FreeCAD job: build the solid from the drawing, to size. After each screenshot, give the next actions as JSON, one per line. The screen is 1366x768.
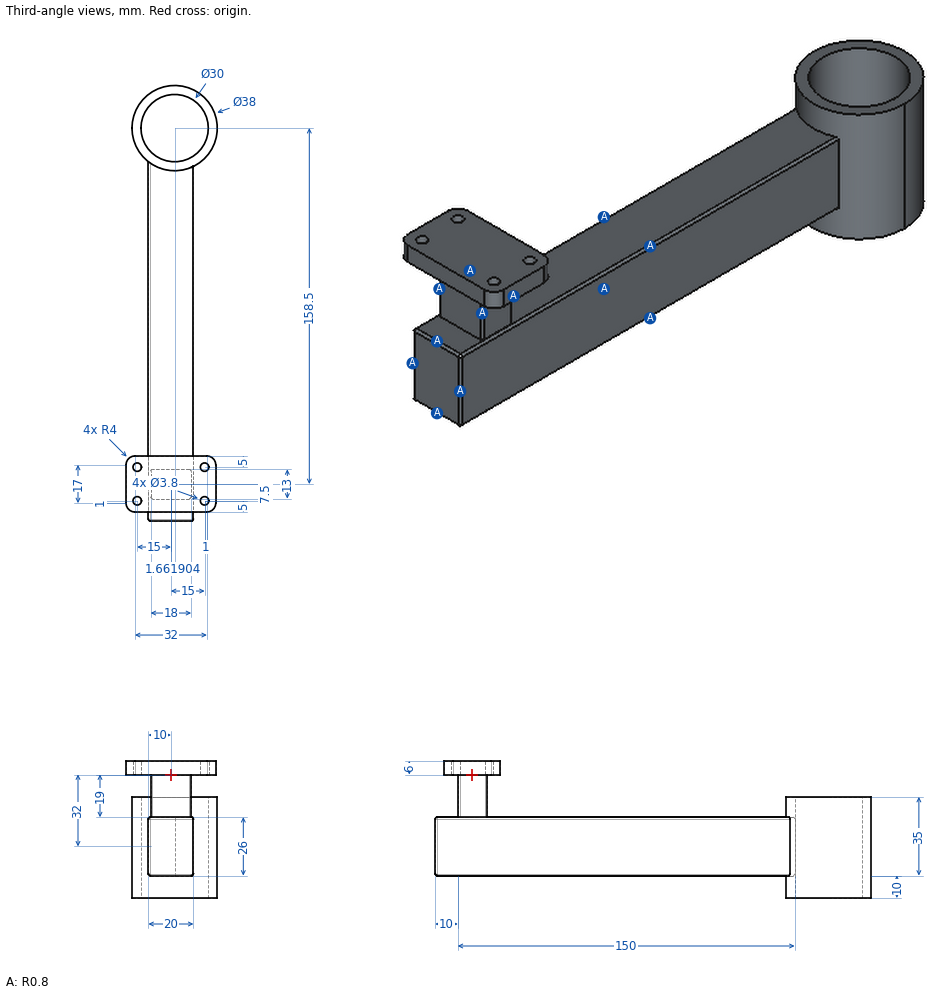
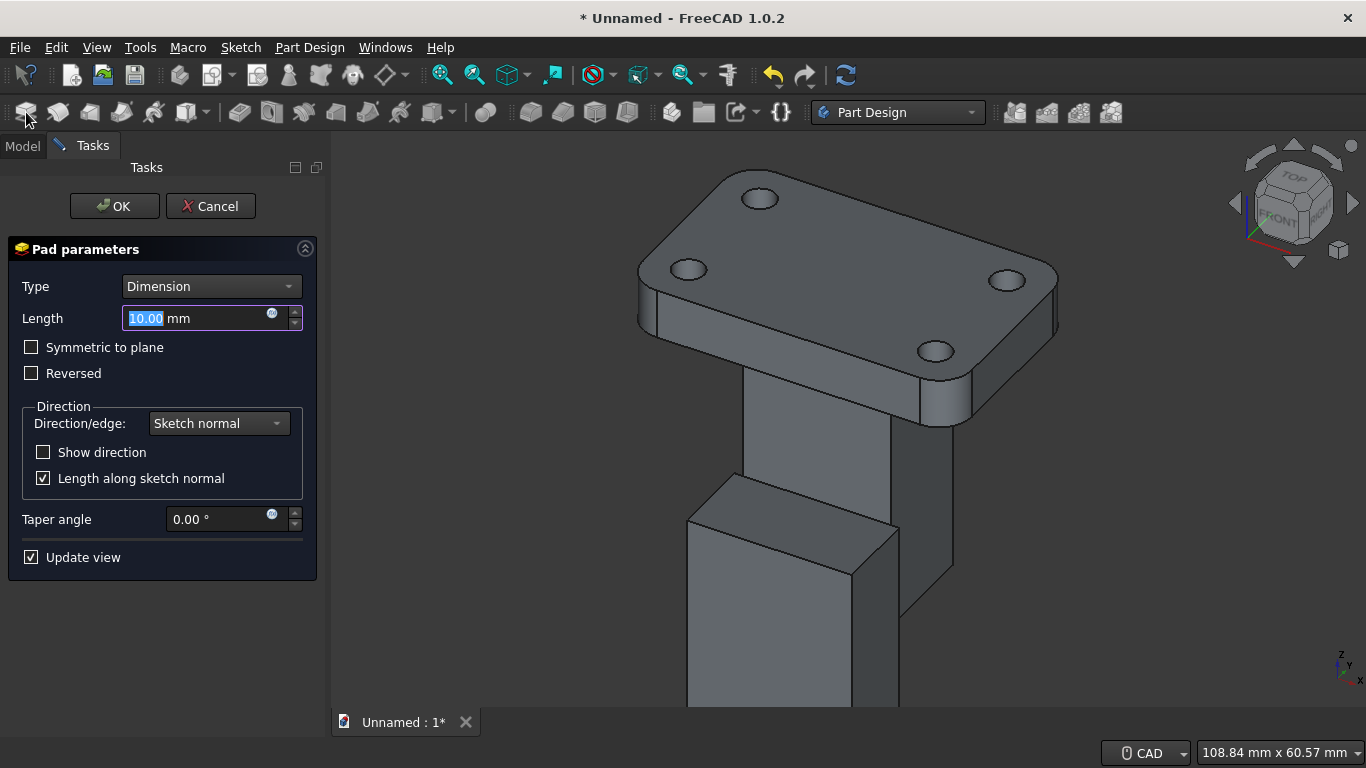
{"action": "left_click", "coordinate": [212, 286]}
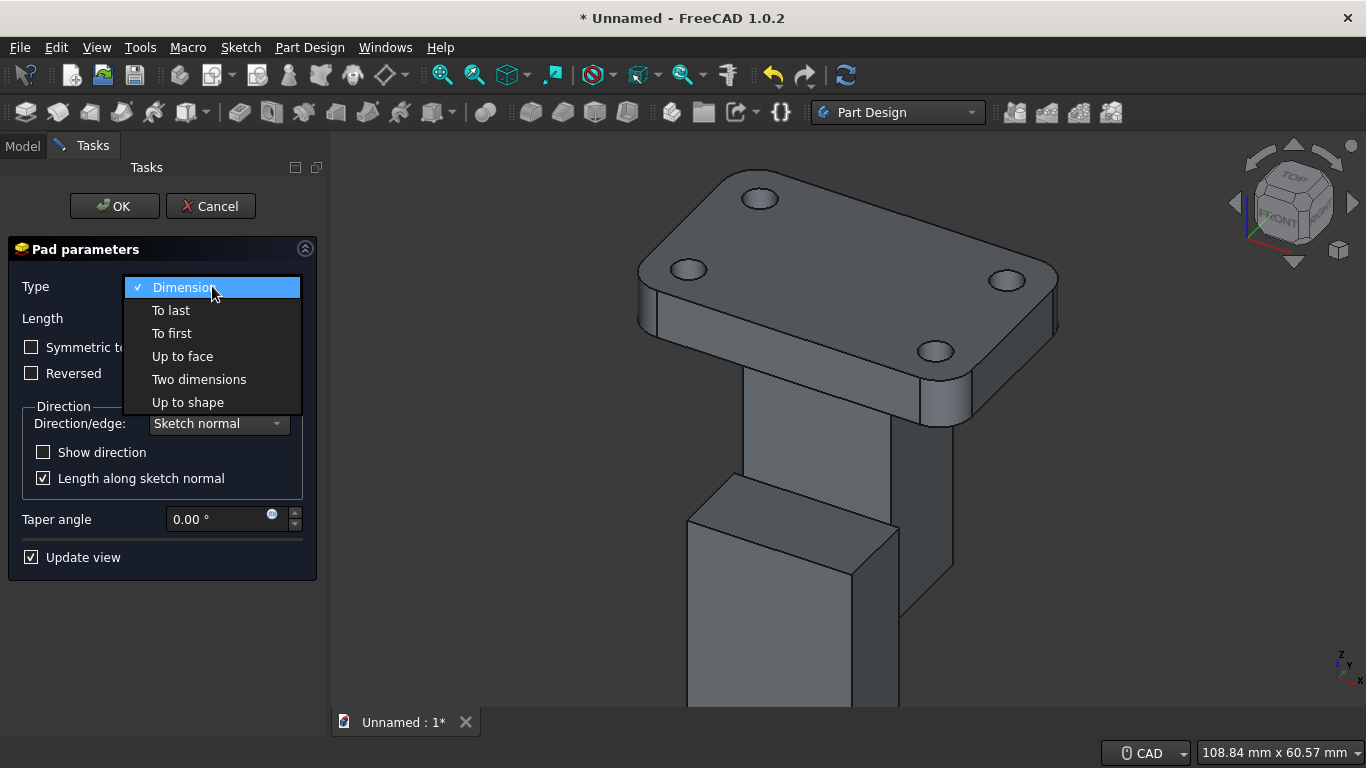
{"action": "left_click", "coordinate": [212, 380]}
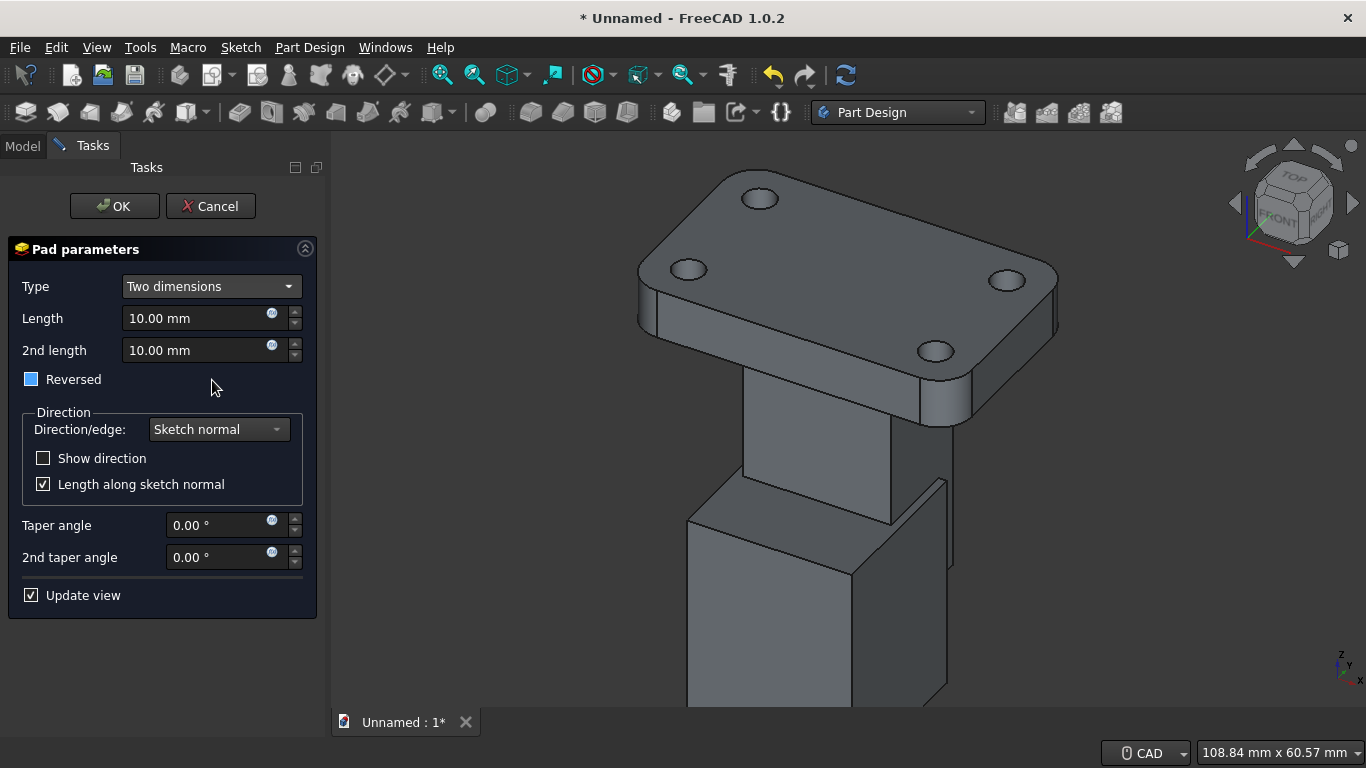
{"action": "triple_click", "coordinate": [204, 318]}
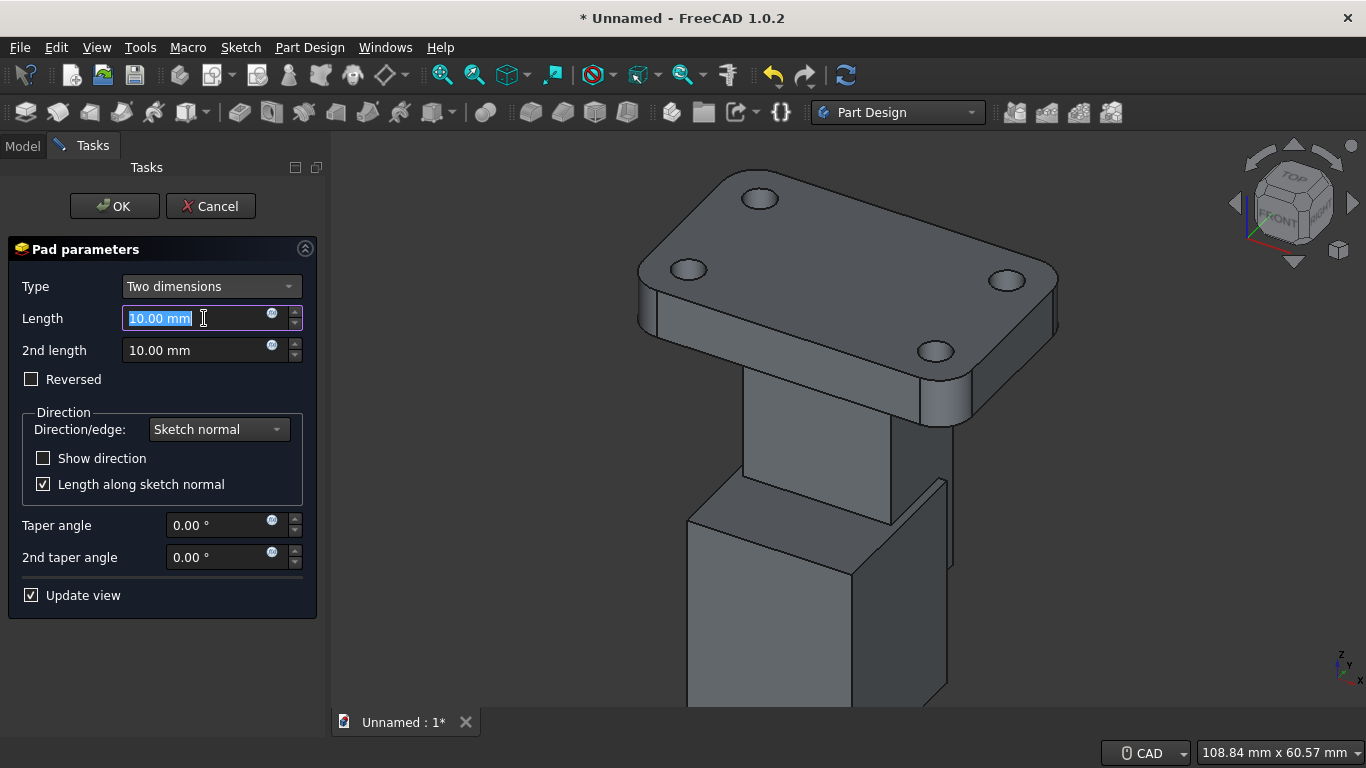
{"action": "type", "text": "10"}
{"action": "key", "text": "Tab"}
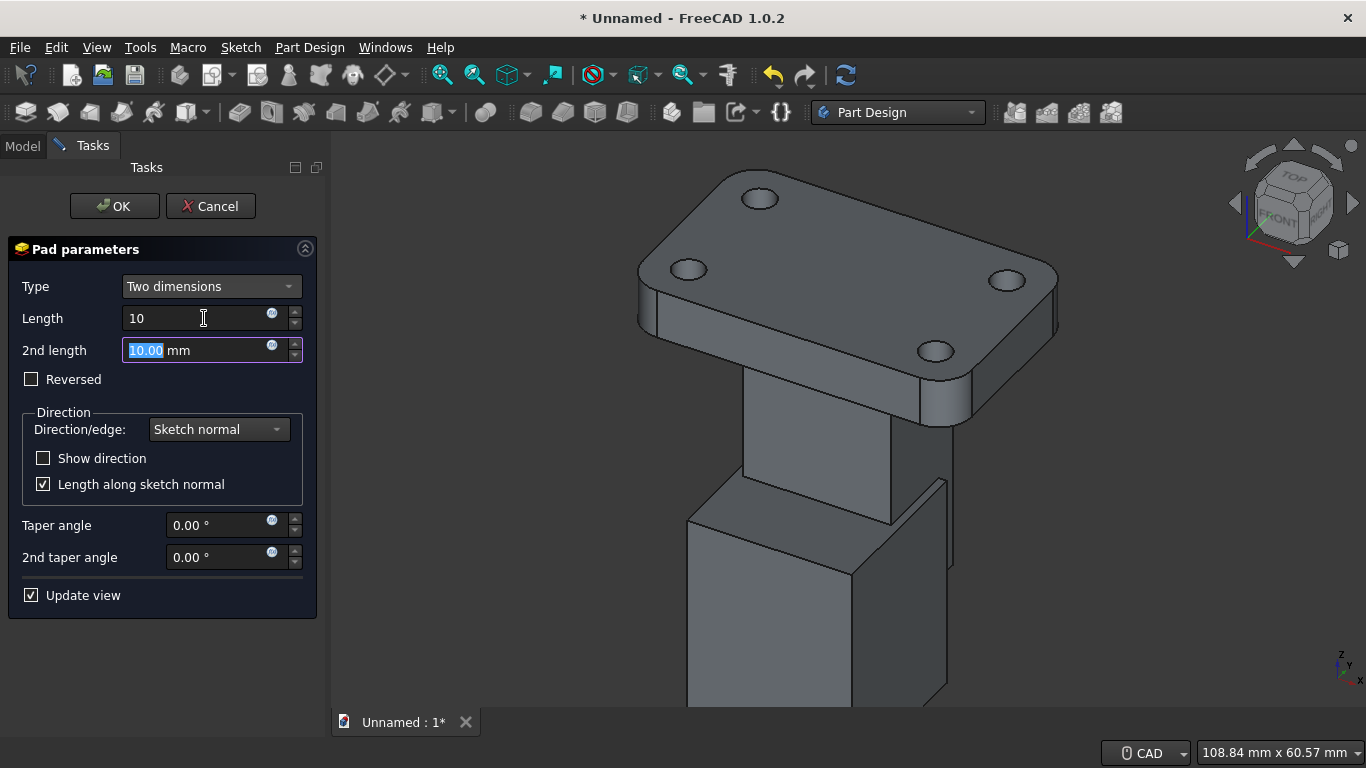
{"action": "type", "text": "150"}
{"action": "key", "text": "Tab"}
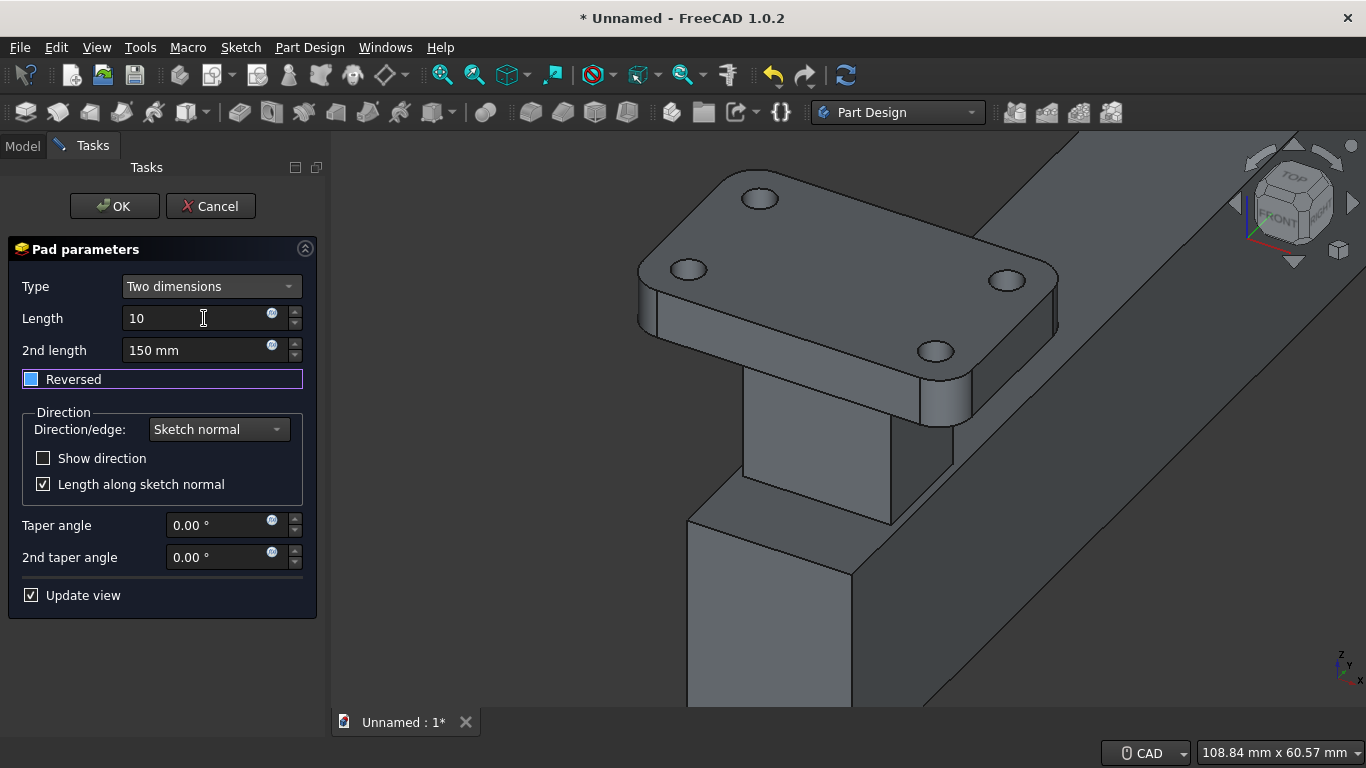
{"action": "left_click", "coordinate": [115, 206]}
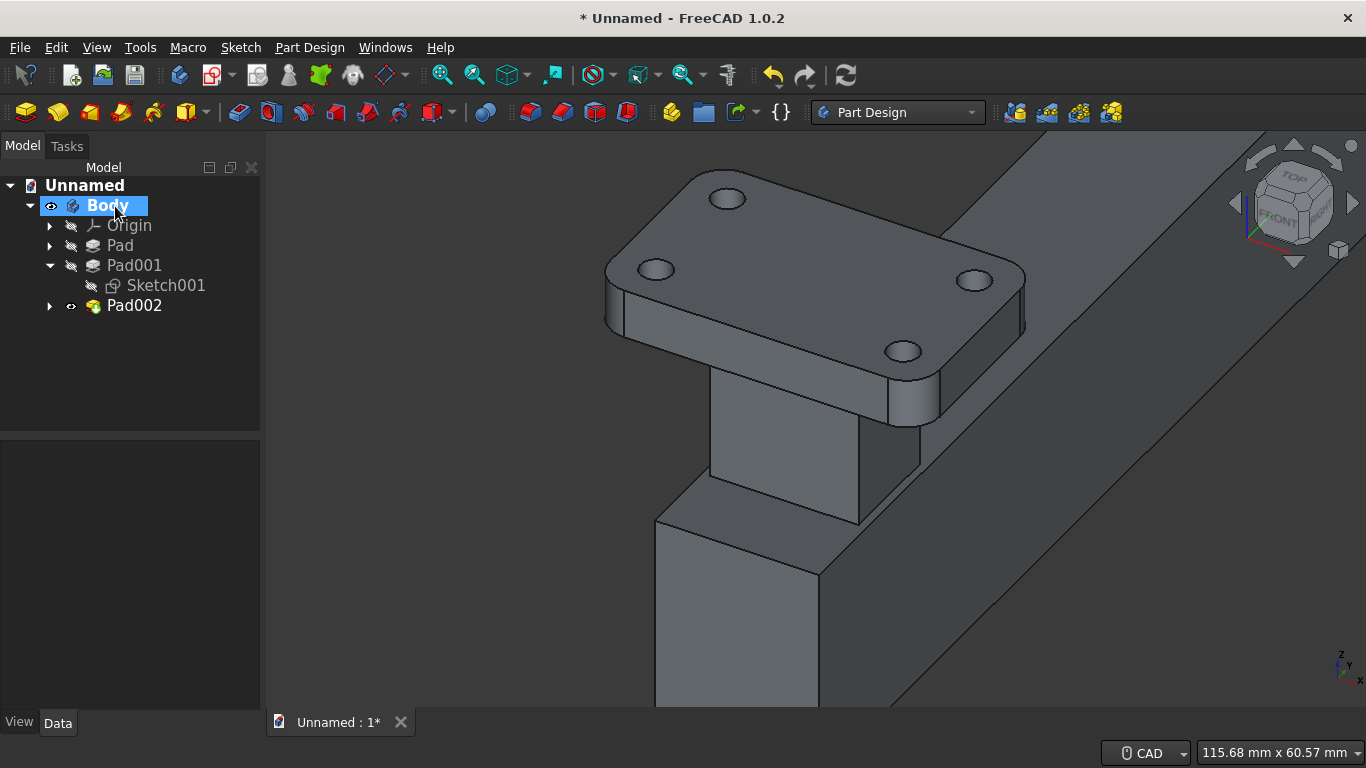
{"action": "left_click", "coordinate": [444, 76]}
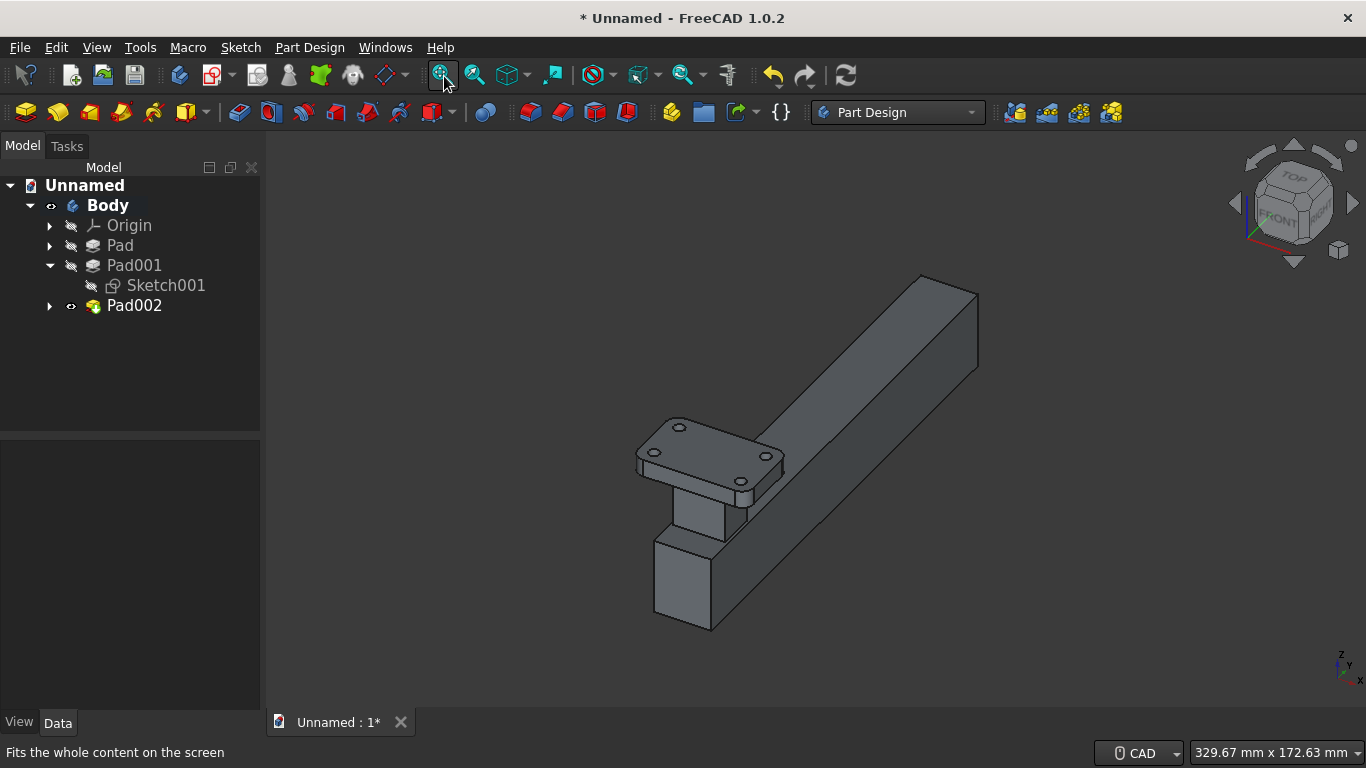
{"action": "key", "text": "5"}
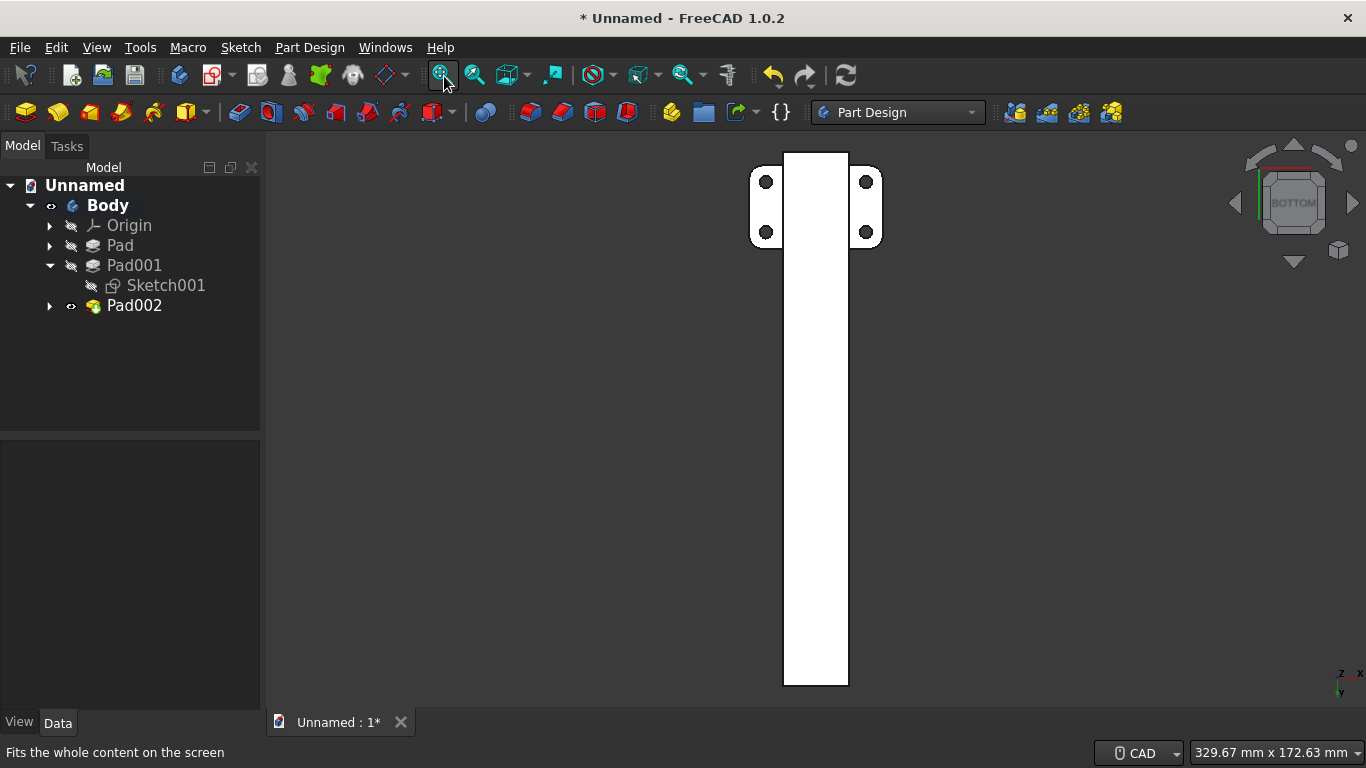
{"action": "left_click", "coordinate": [816, 647]}